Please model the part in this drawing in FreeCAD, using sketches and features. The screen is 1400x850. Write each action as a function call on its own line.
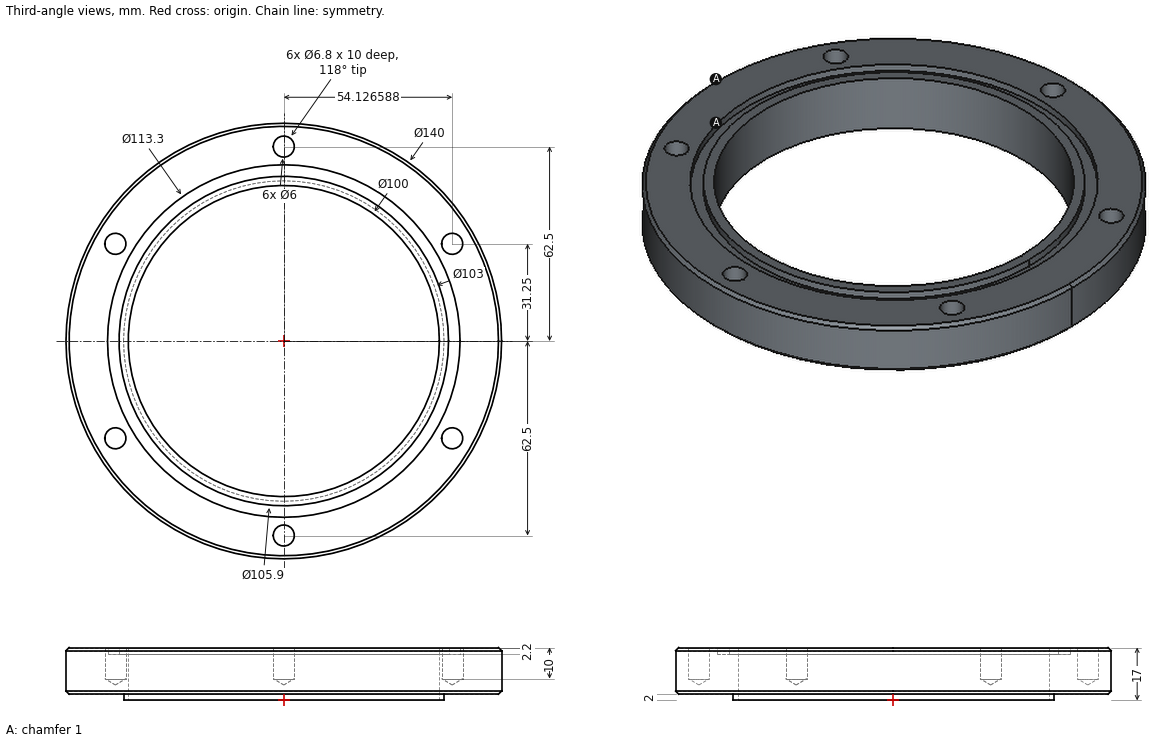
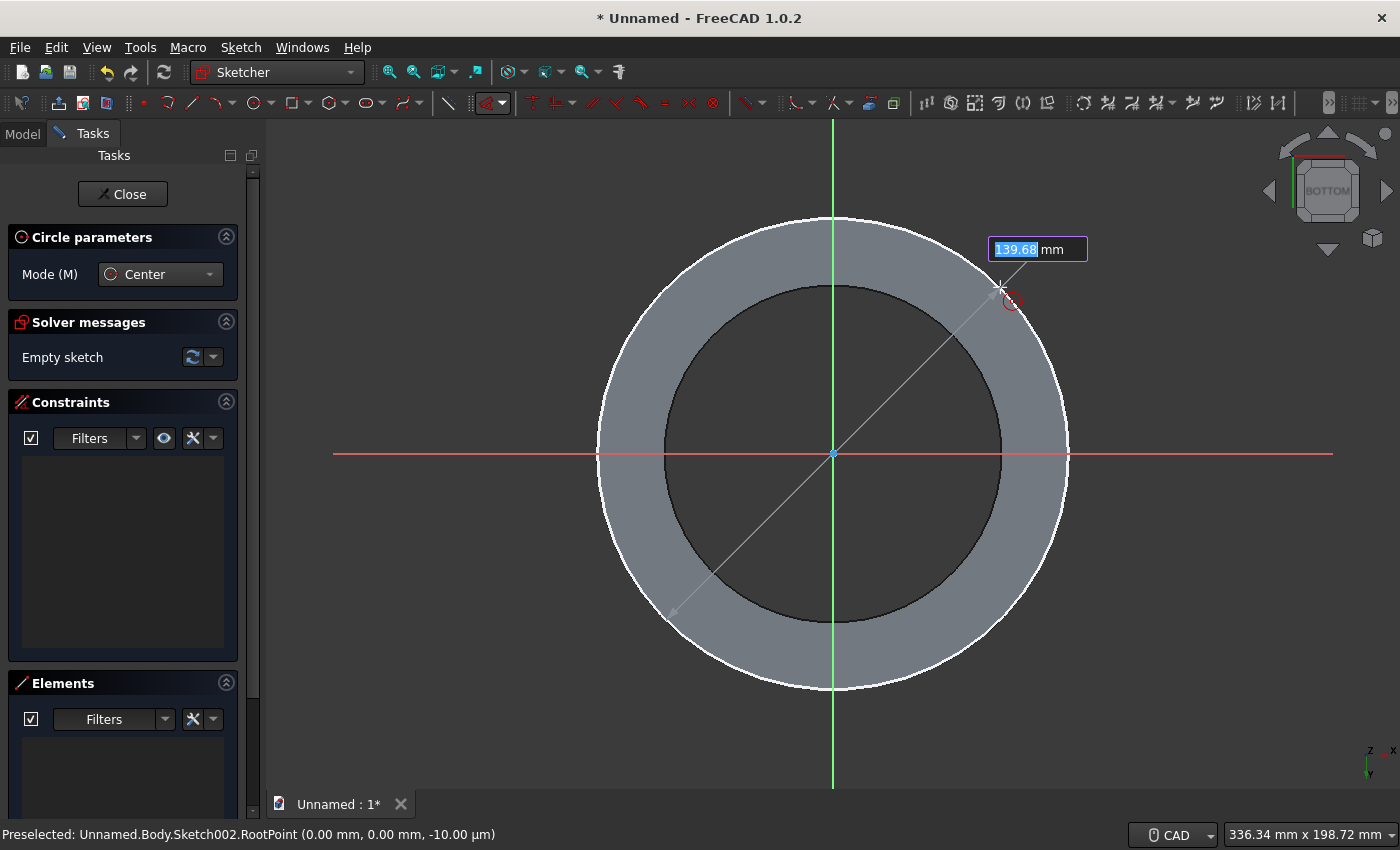
text(140)
key(Return)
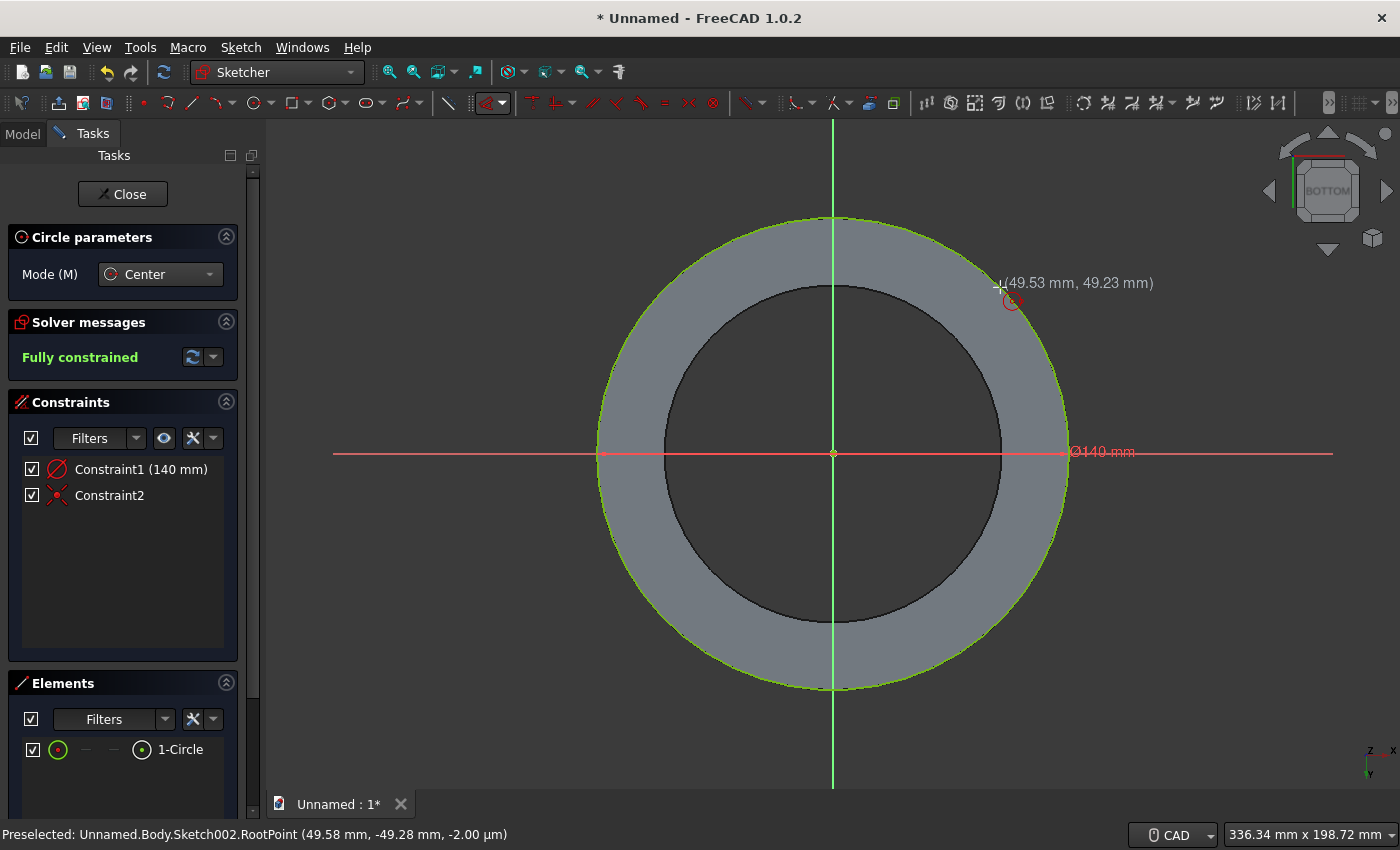
click(833, 454)
move(956, 331)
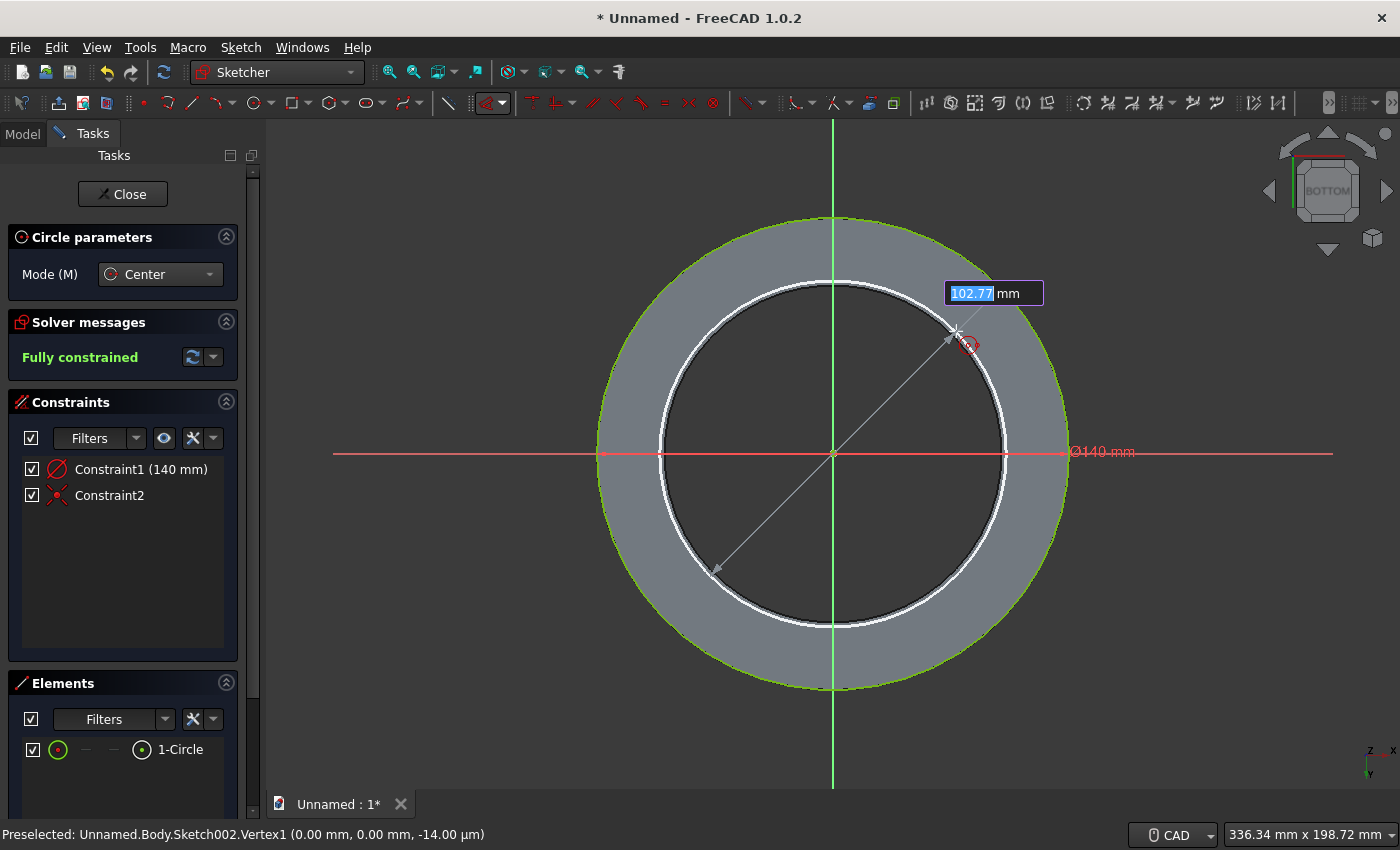
text(103)
key(Return)
key(Escape)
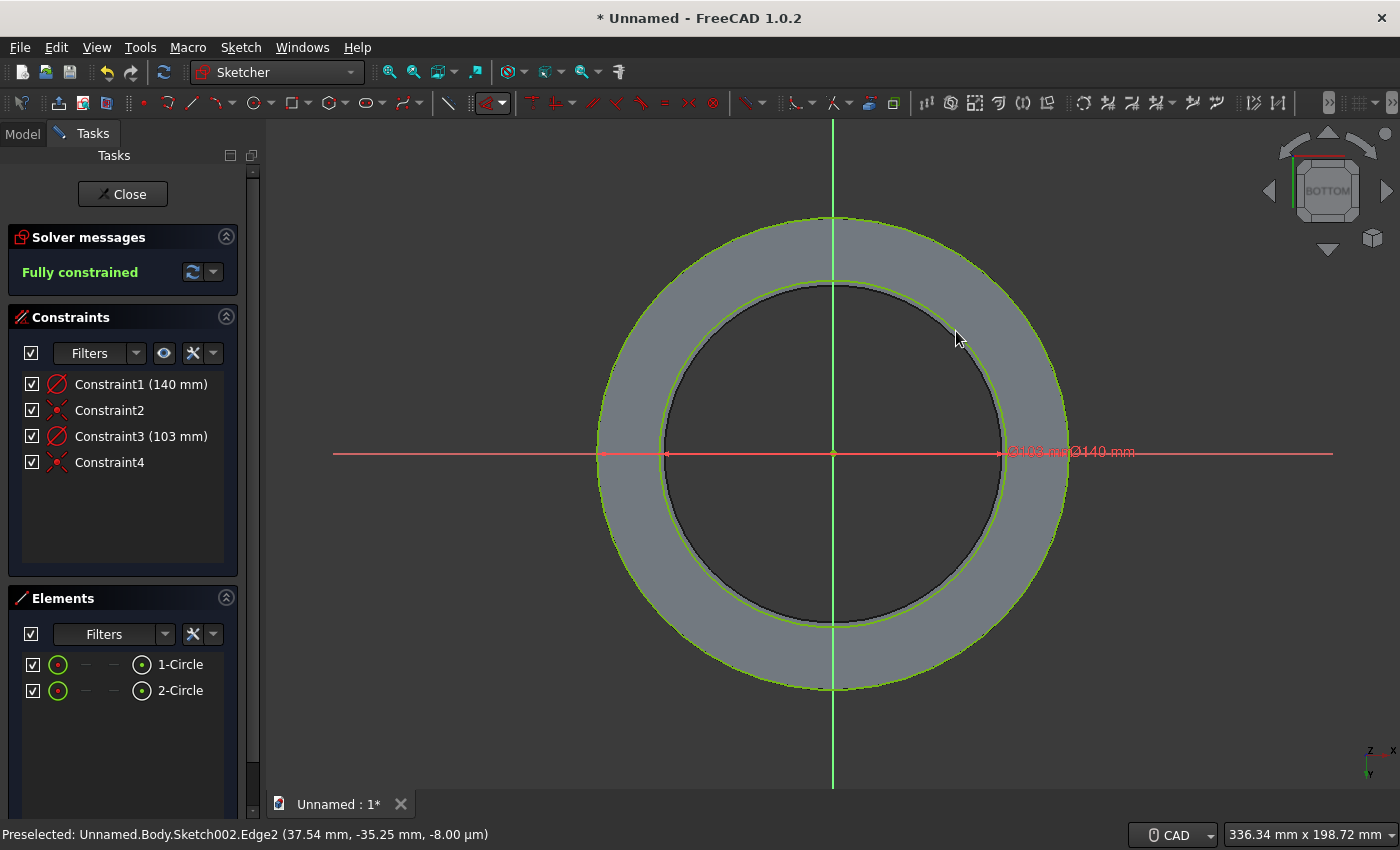
click(123, 194)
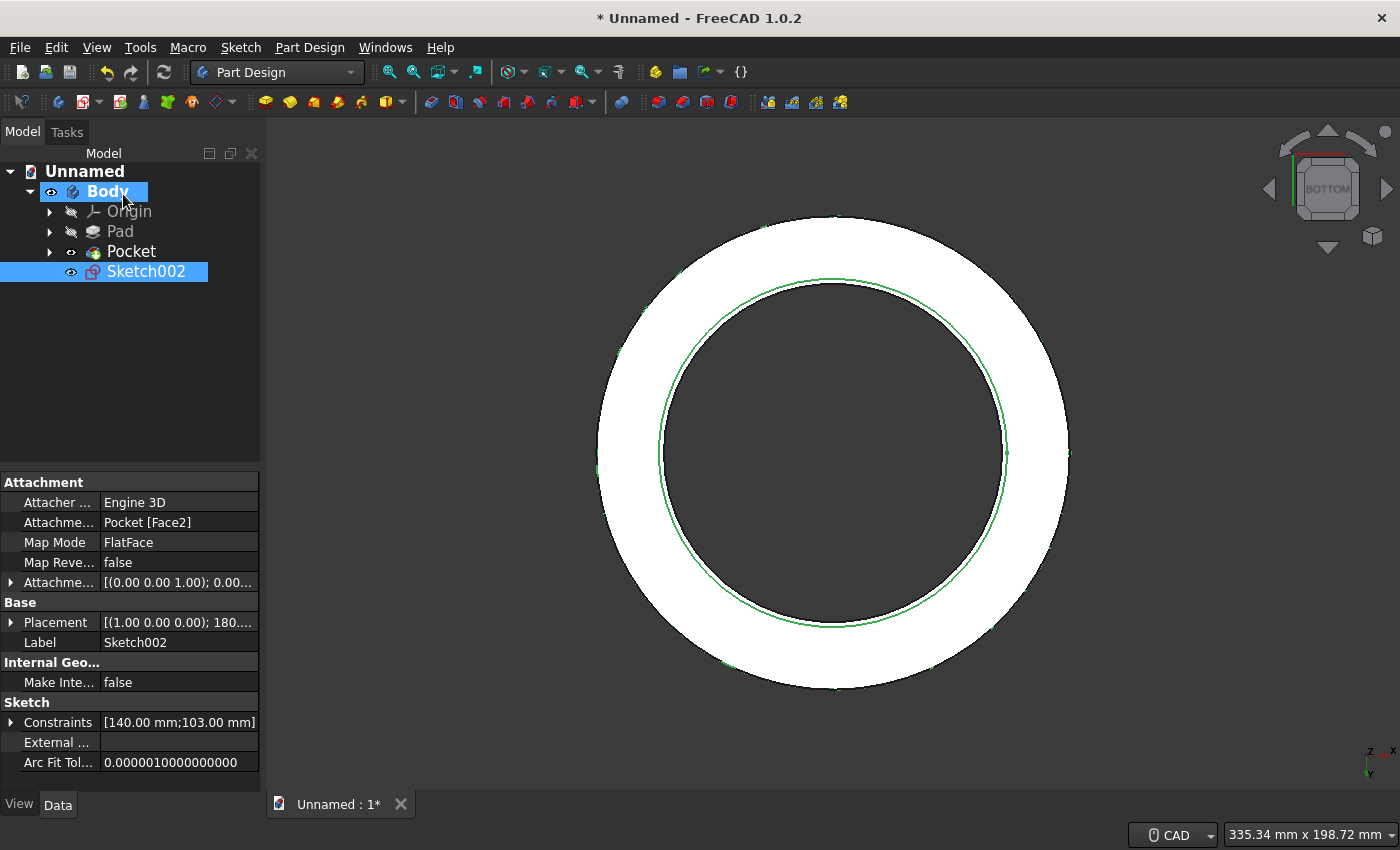
click(432, 102)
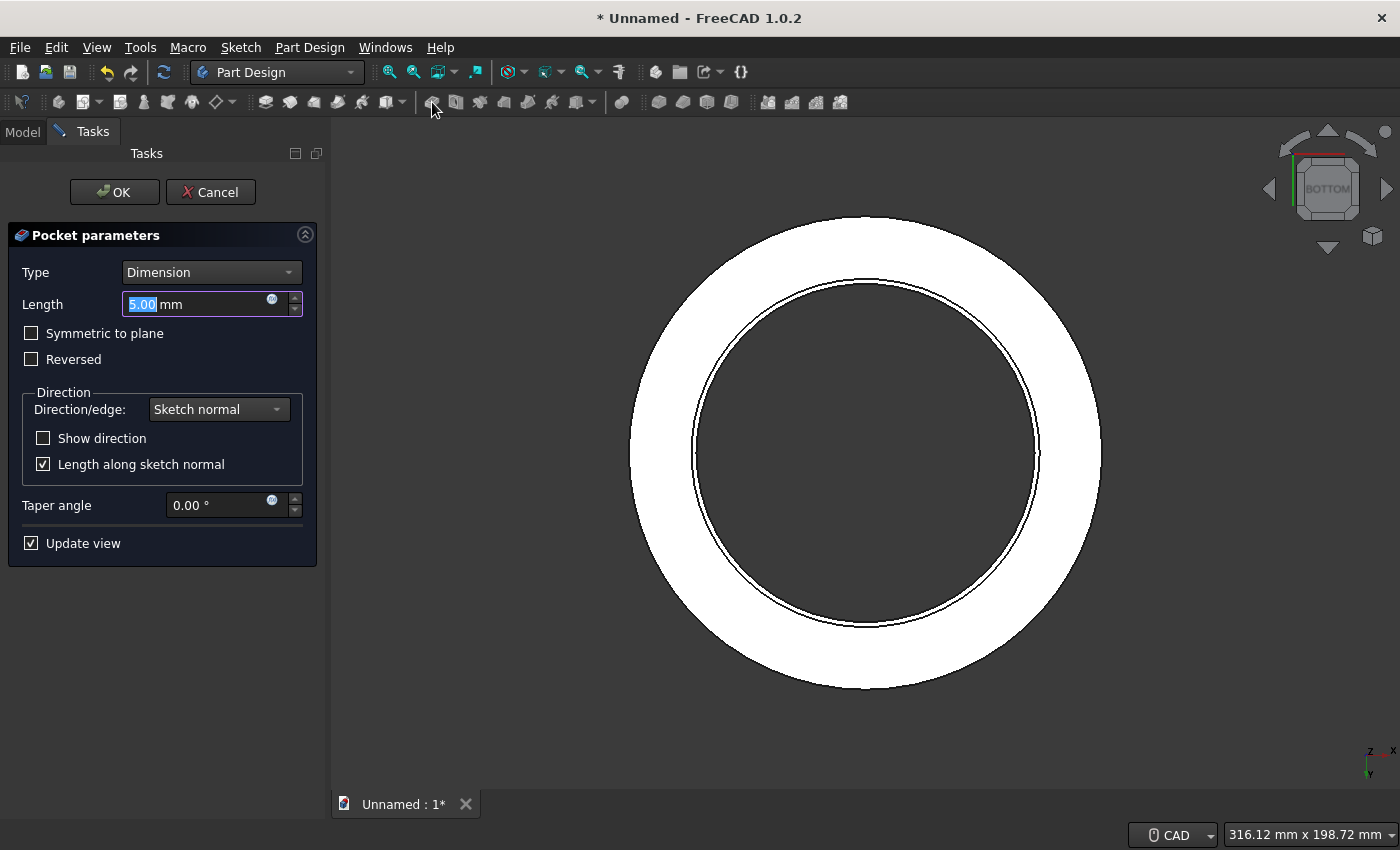
text(2)
key(Tab)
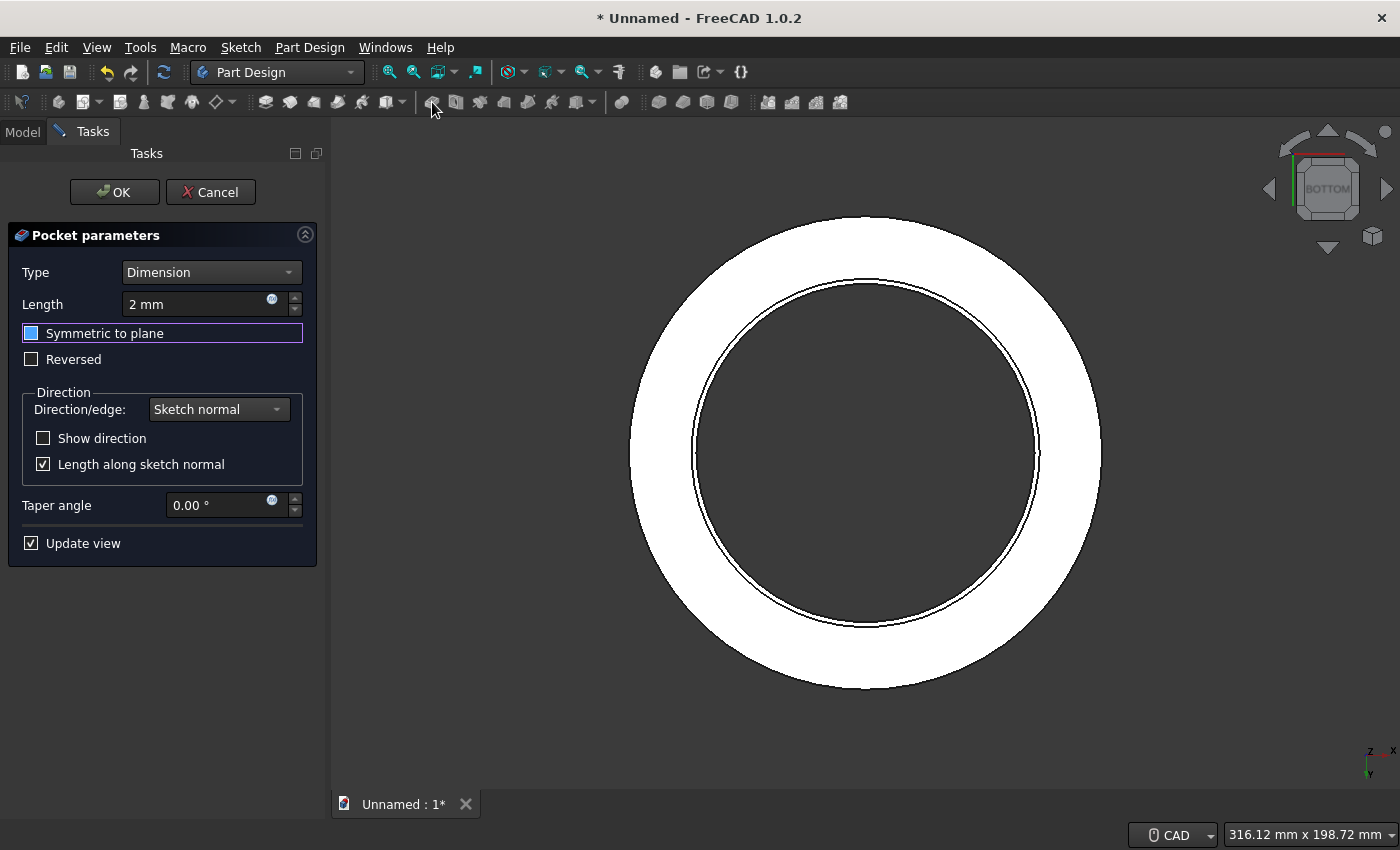
click(115, 192)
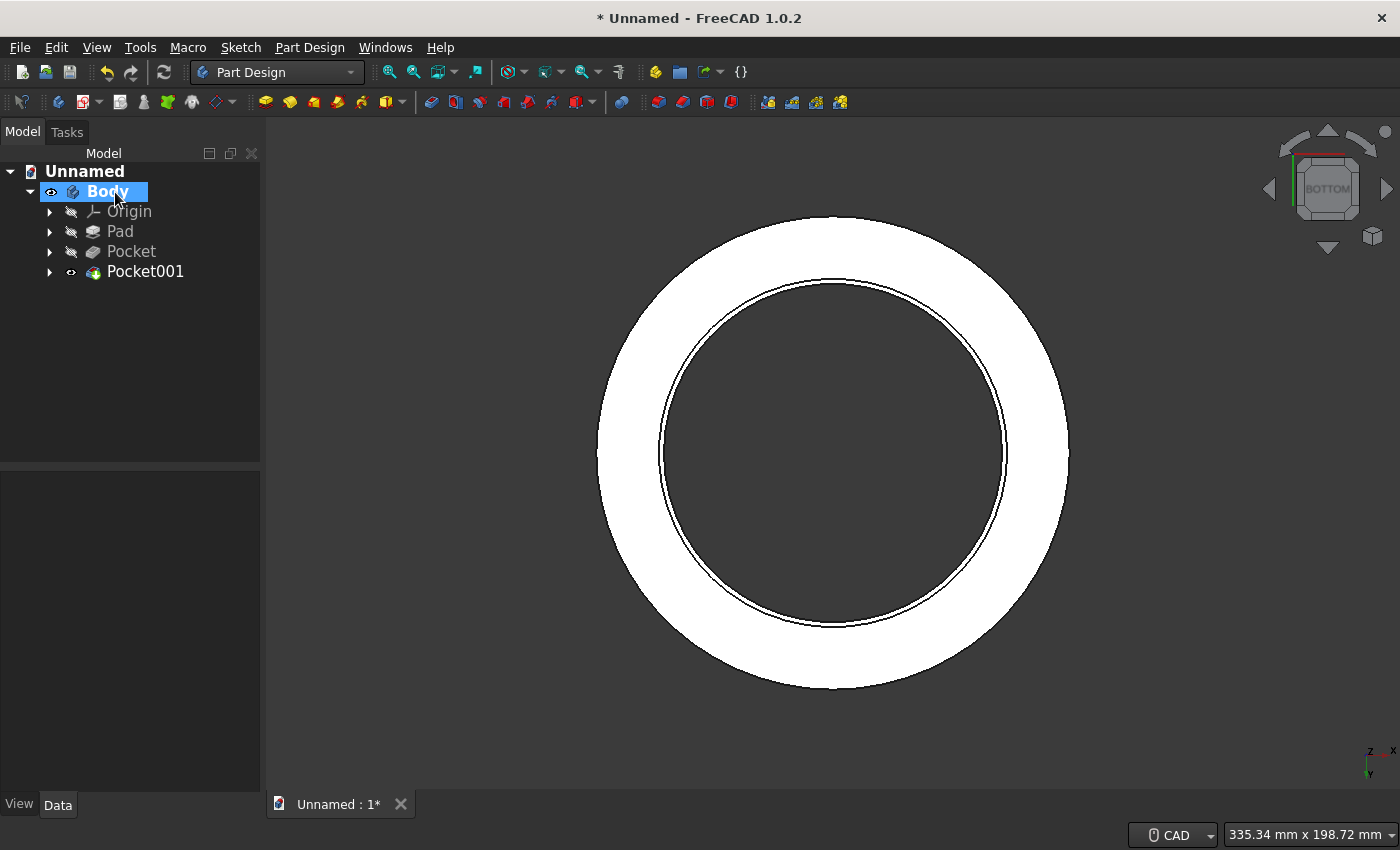
key(0)